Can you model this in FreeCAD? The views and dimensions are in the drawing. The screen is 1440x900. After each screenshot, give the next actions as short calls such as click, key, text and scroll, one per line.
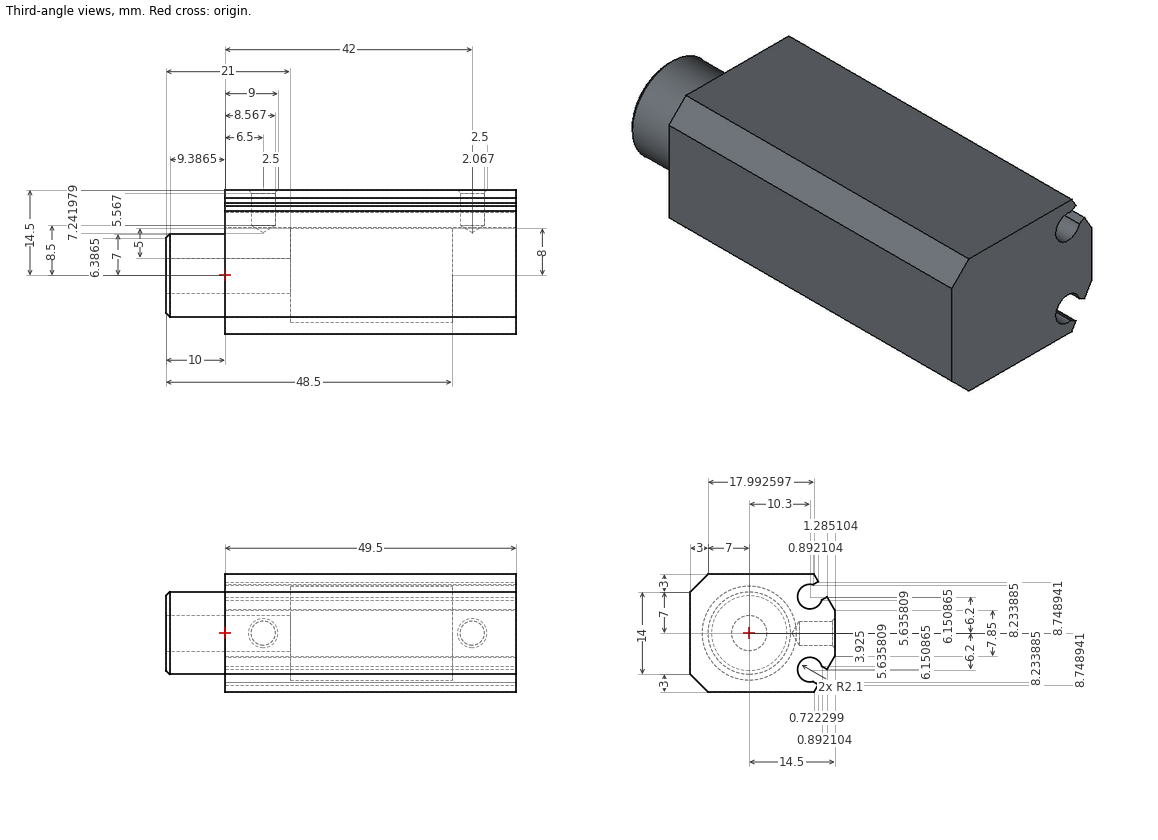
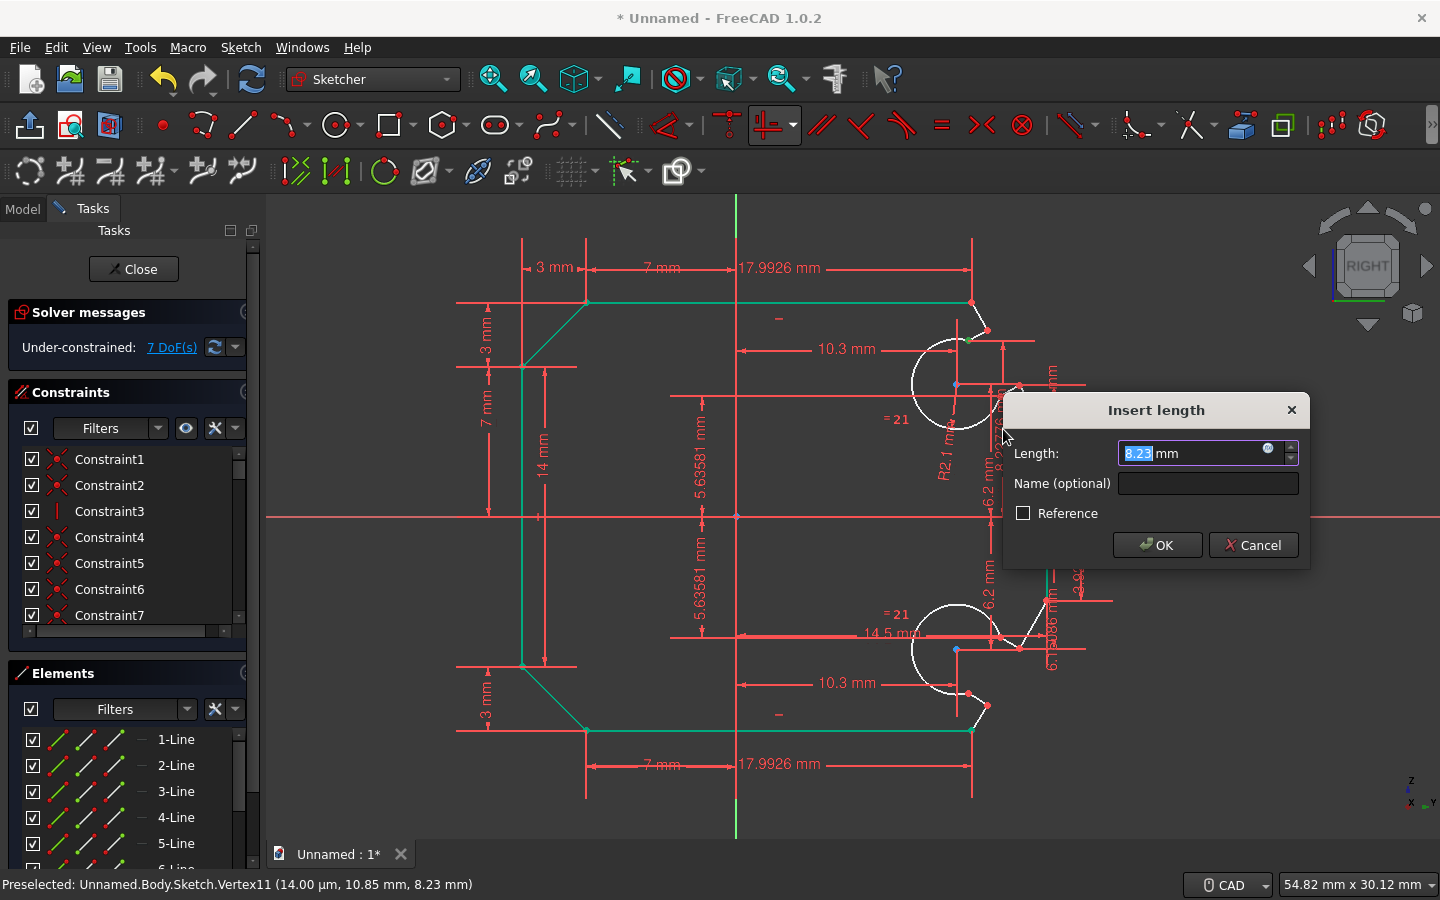
text(8.233885)
key(Return)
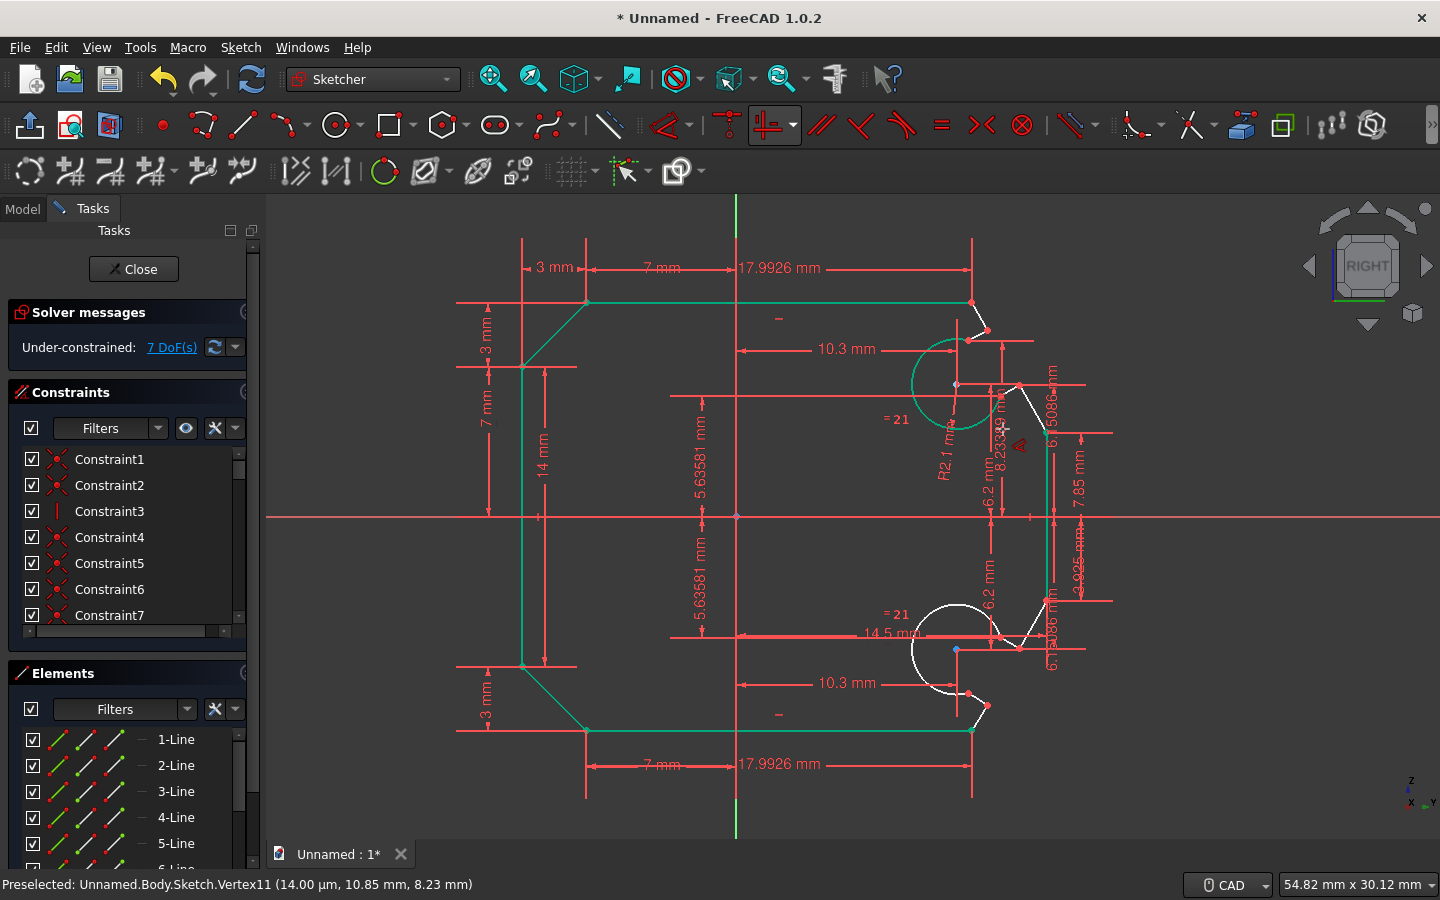
click(988, 330)
click(1022, 358)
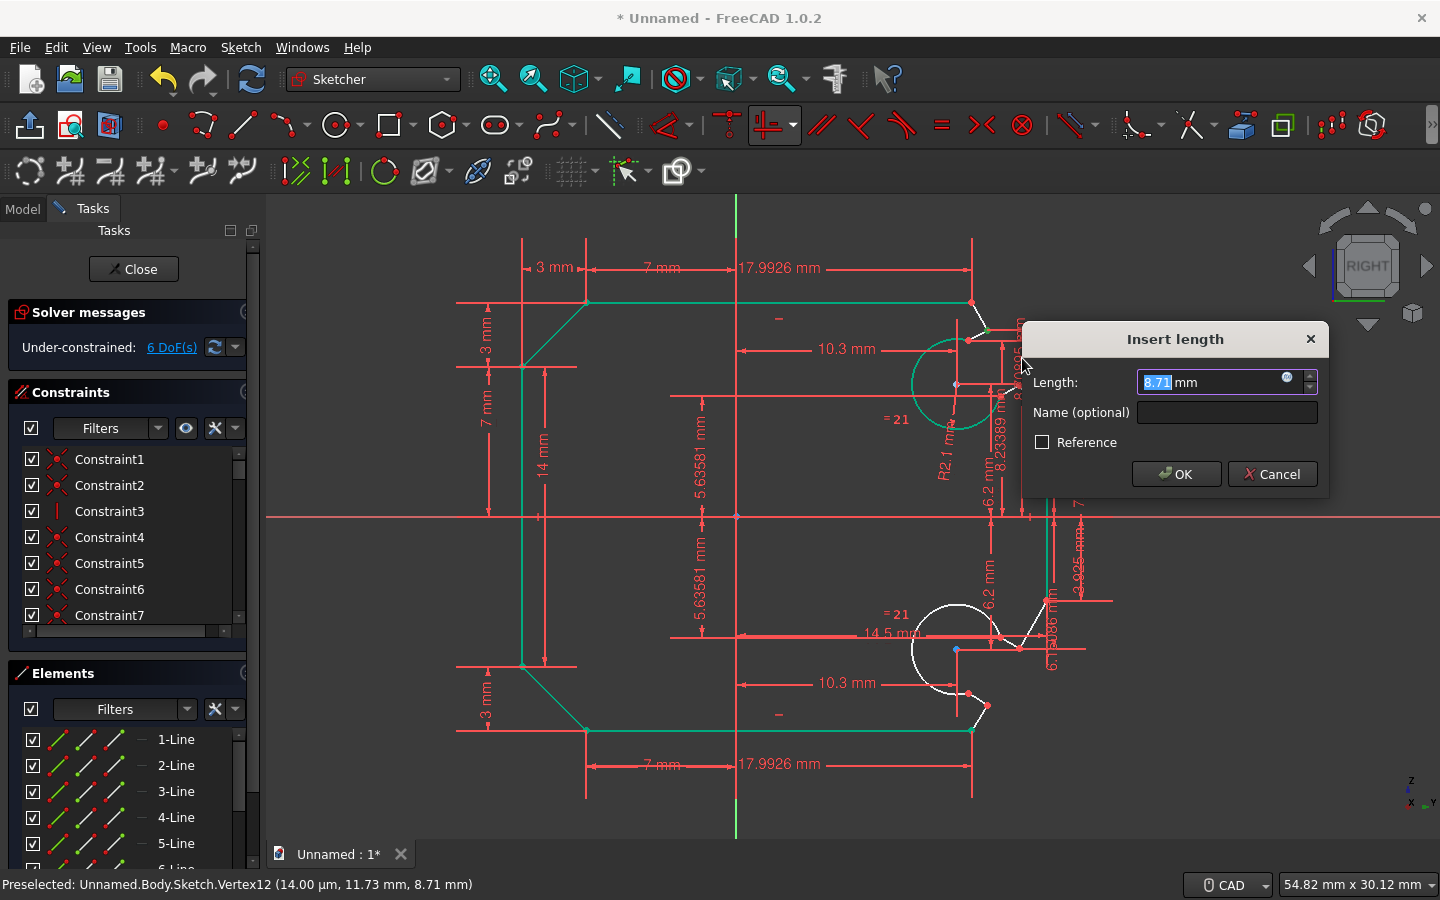
text(8.748941)
key(Return)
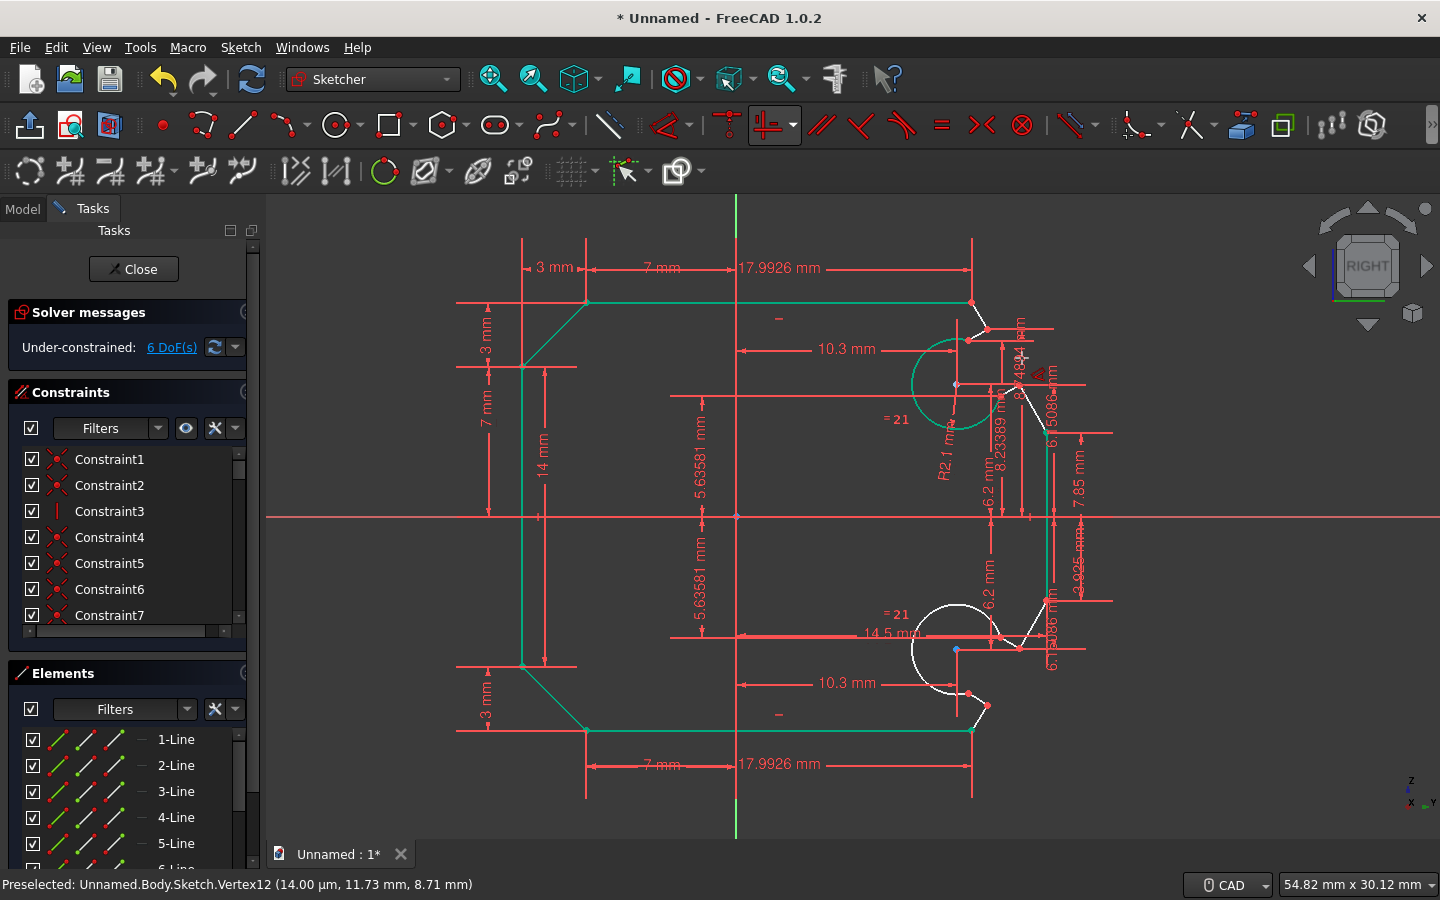
click(988, 705)
click(1022, 677)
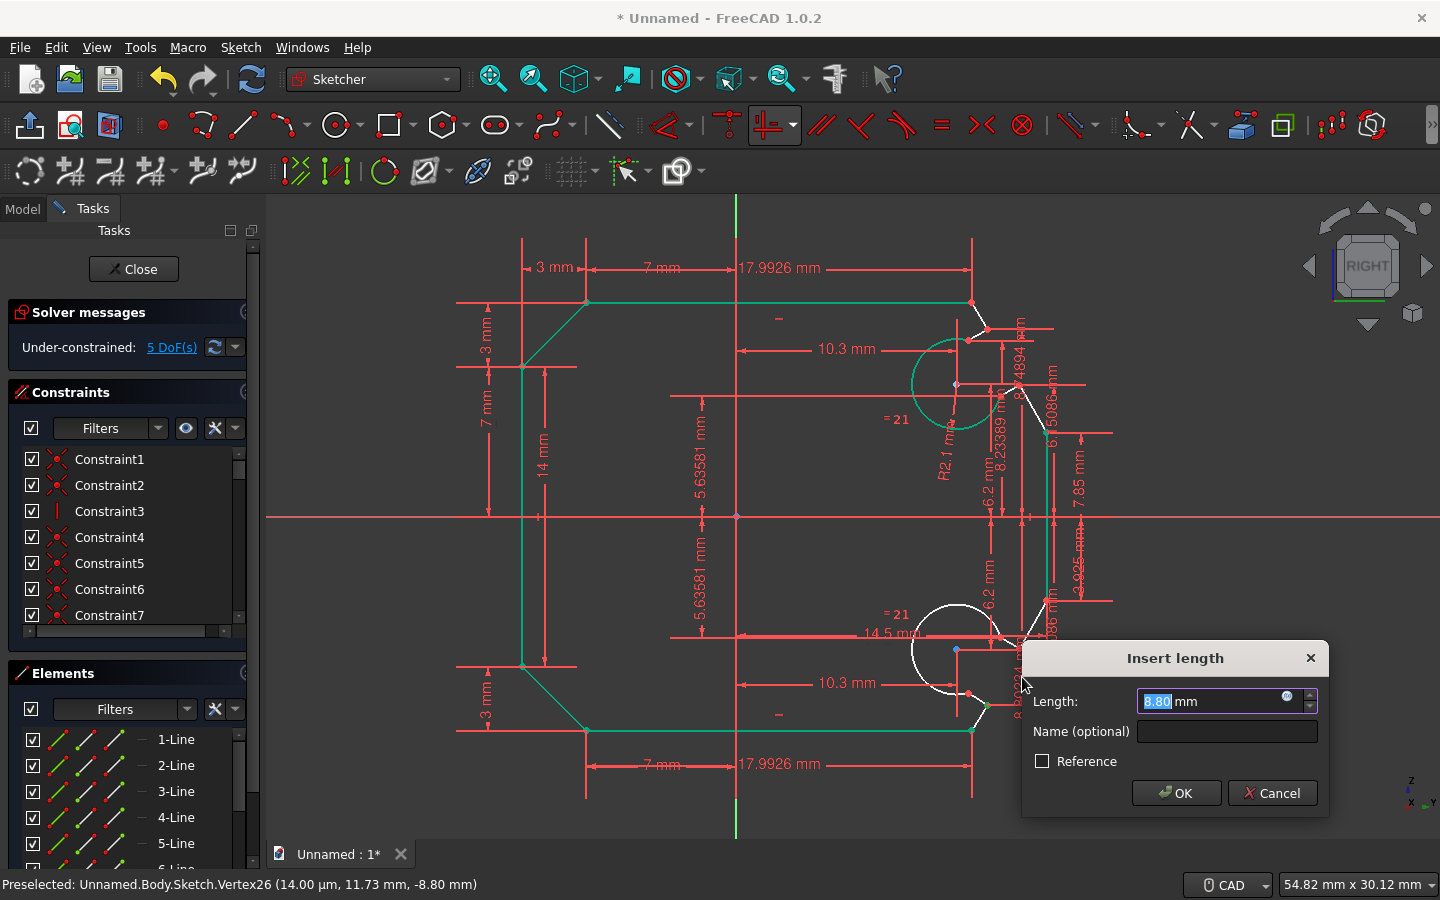
text(8.748941)
key(Return)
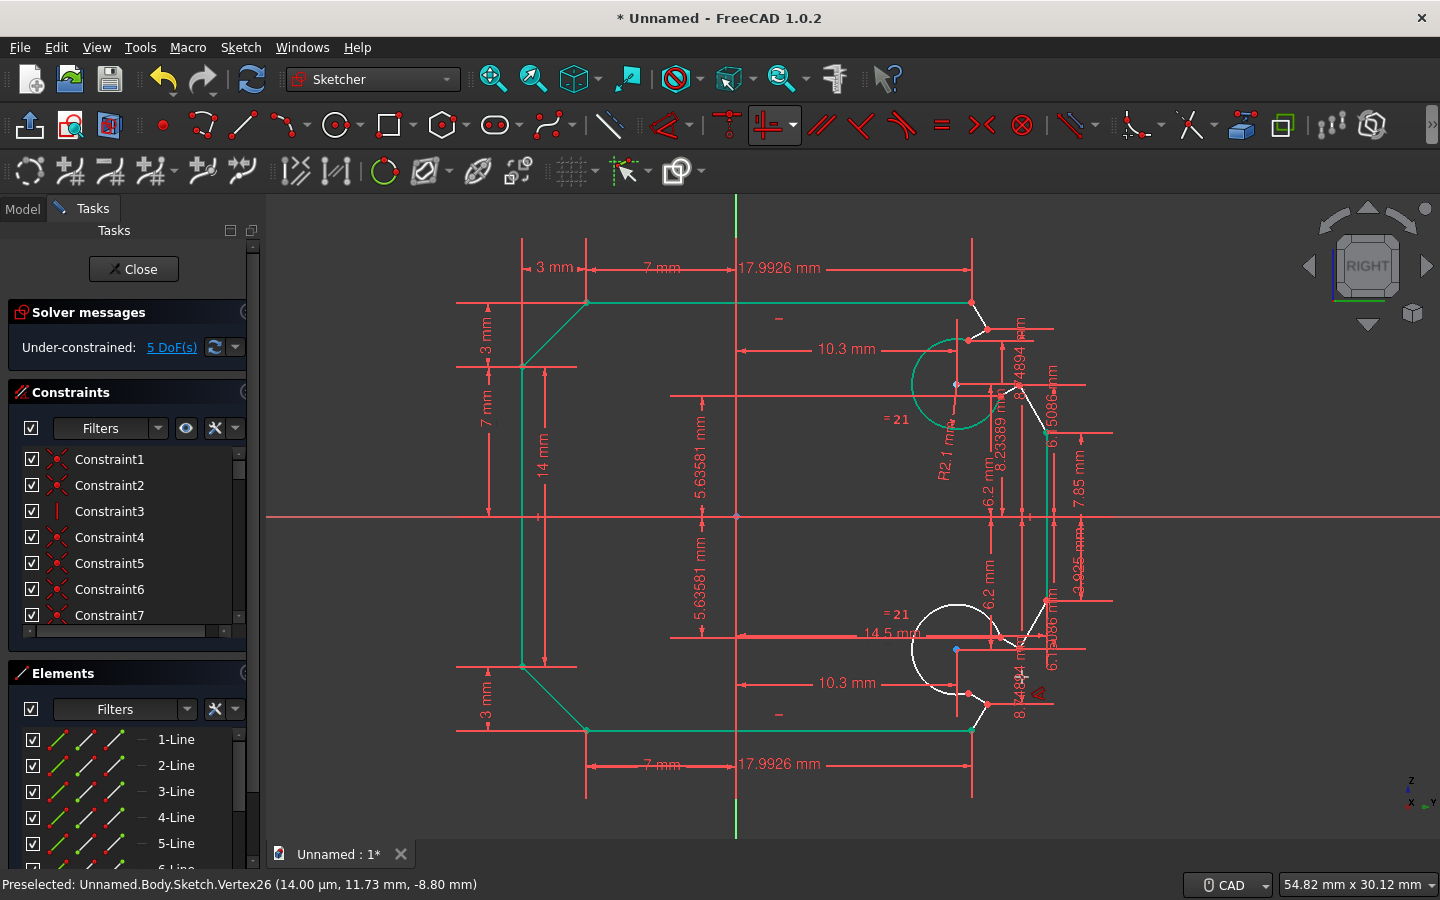
click(969, 693)
click(1003, 605)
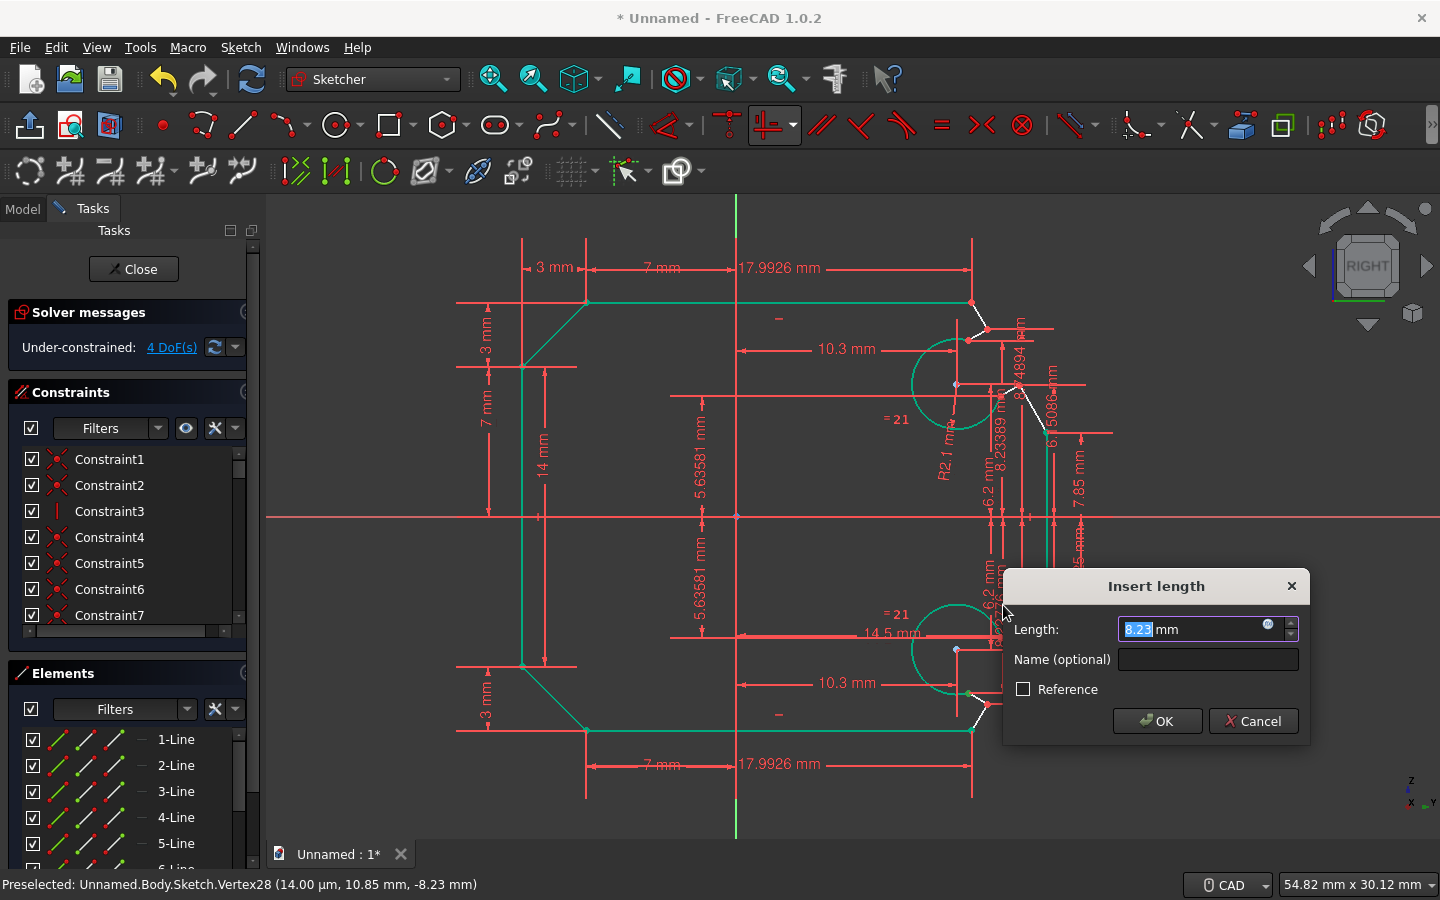
text(8.233885)
key(Return)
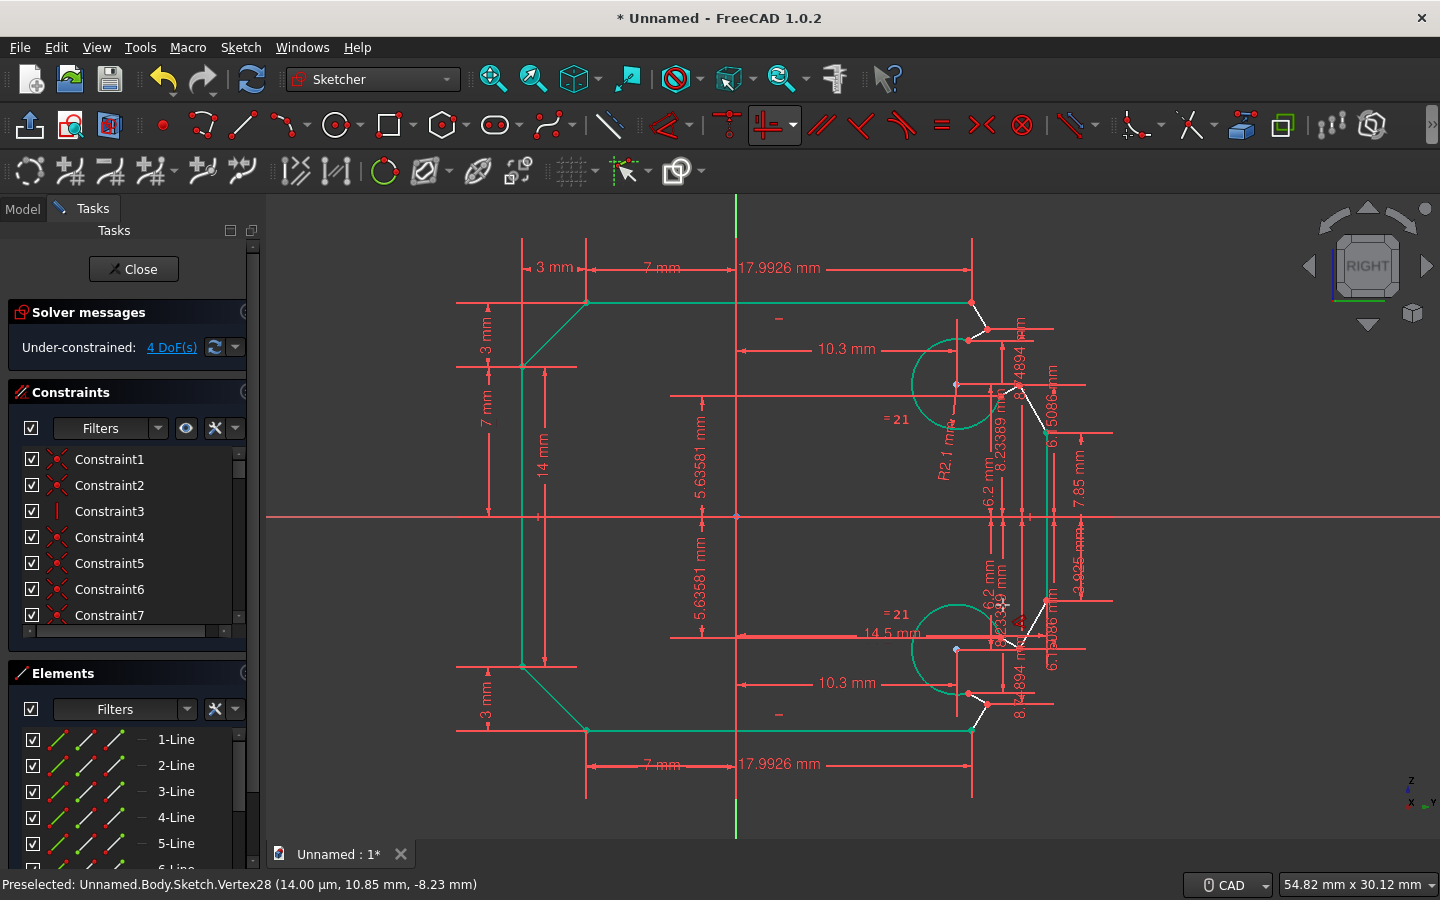
scroll(1010, 643, up, 4)